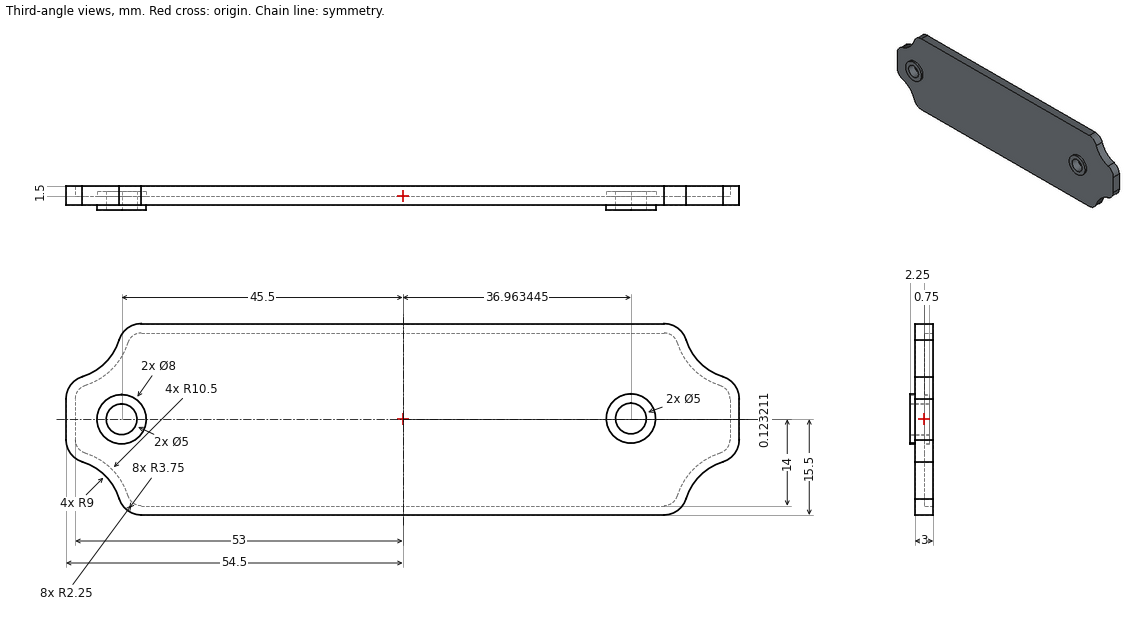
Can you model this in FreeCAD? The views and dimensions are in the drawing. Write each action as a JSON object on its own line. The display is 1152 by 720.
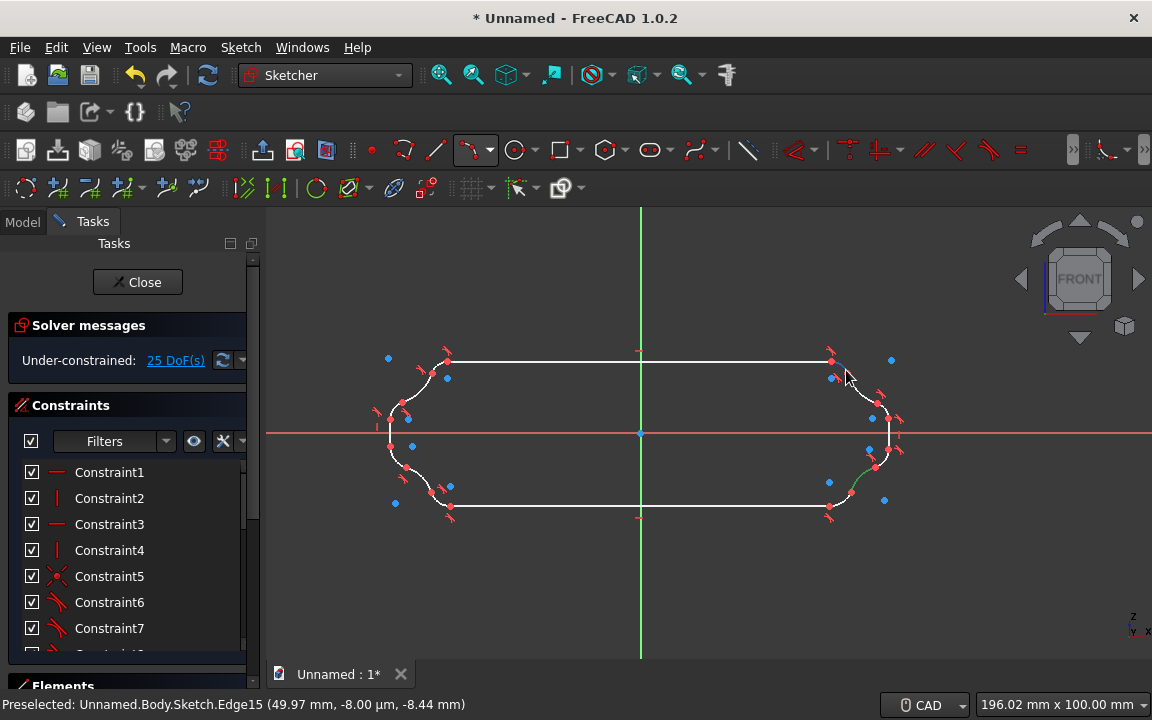
{"action": "scroll", "coordinate": [838, 505], "scroll_direction": "up", "scroll_amount": 3}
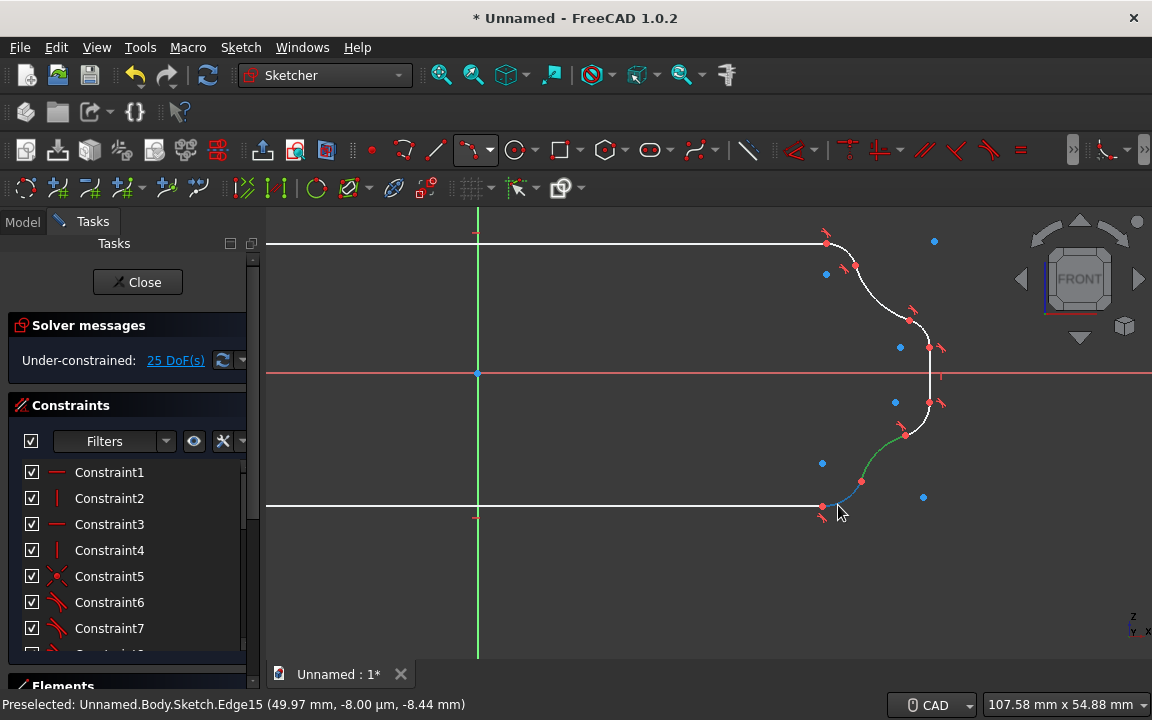
{"action": "left_click", "coordinate": [837, 504]}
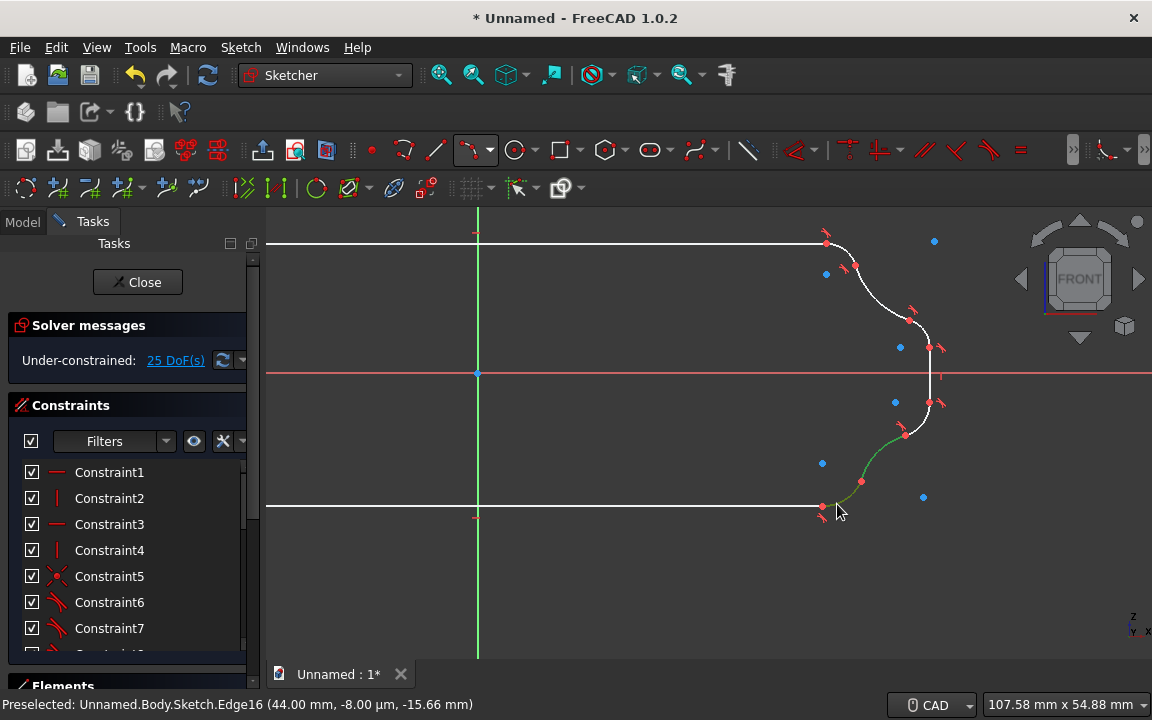
{"action": "left_click", "coordinate": [990, 150]}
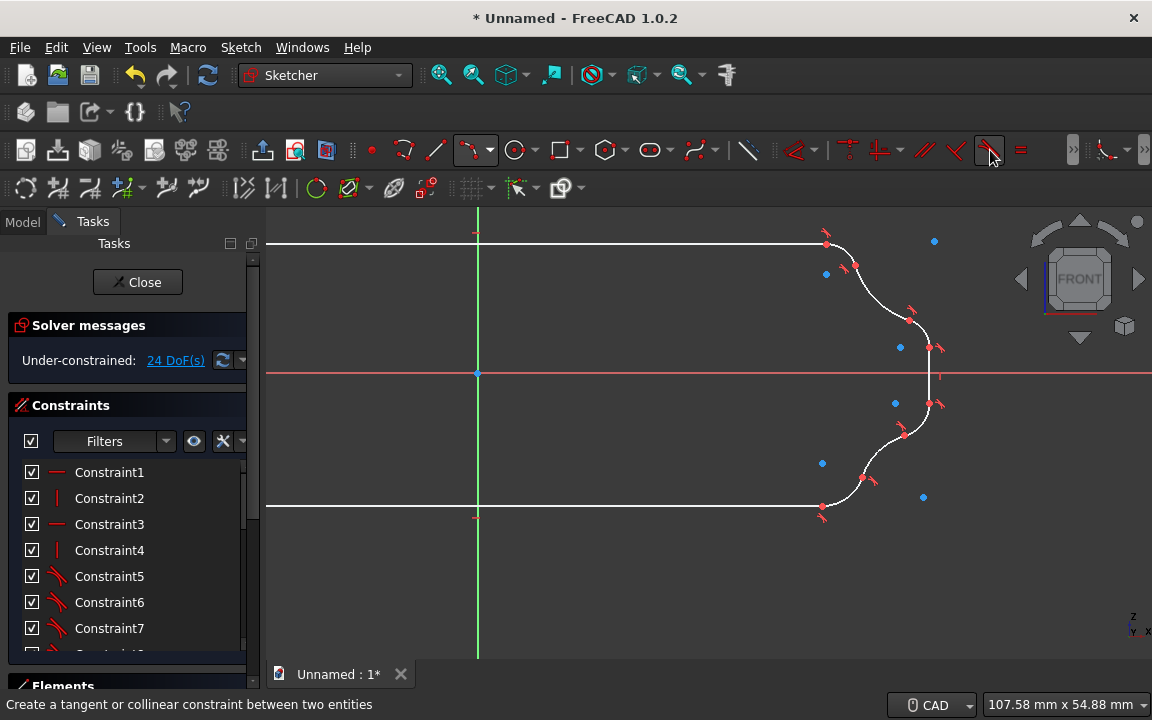
{"action": "scroll", "coordinate": [838, 506], "scroll_direction": "down", "scroll_amount": 3}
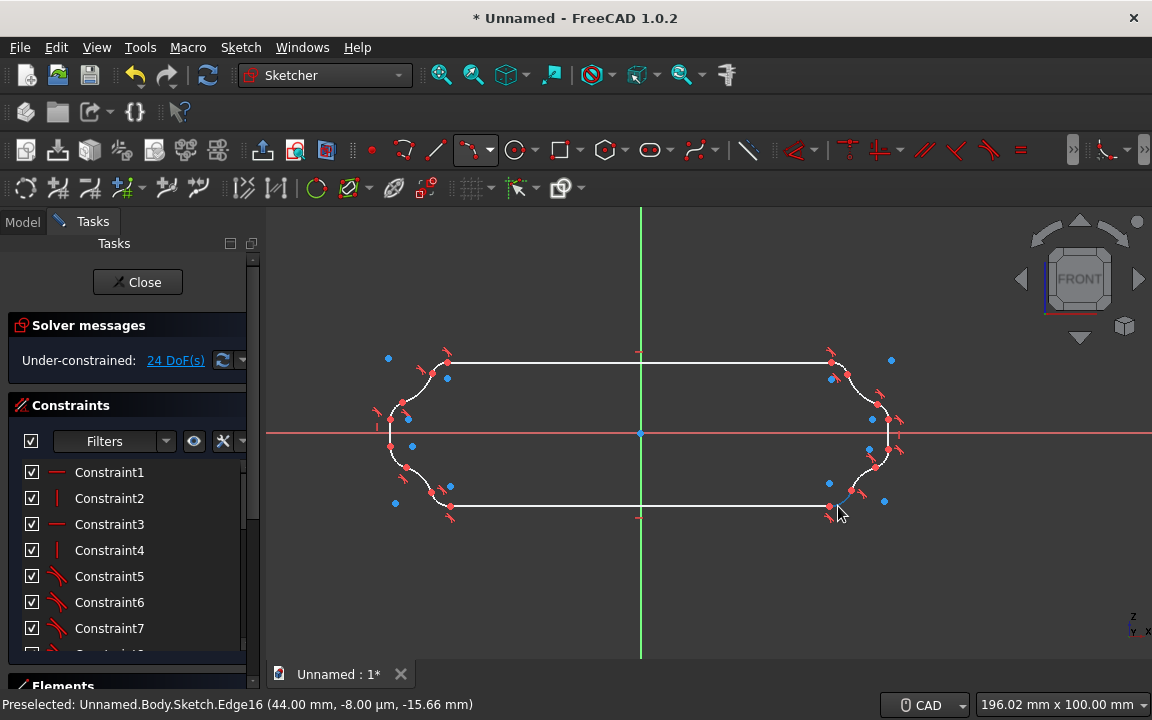
{"action": "scroll", "coordinate": [435, 499], "scroll_direction": "up", "scroll_amount": 4}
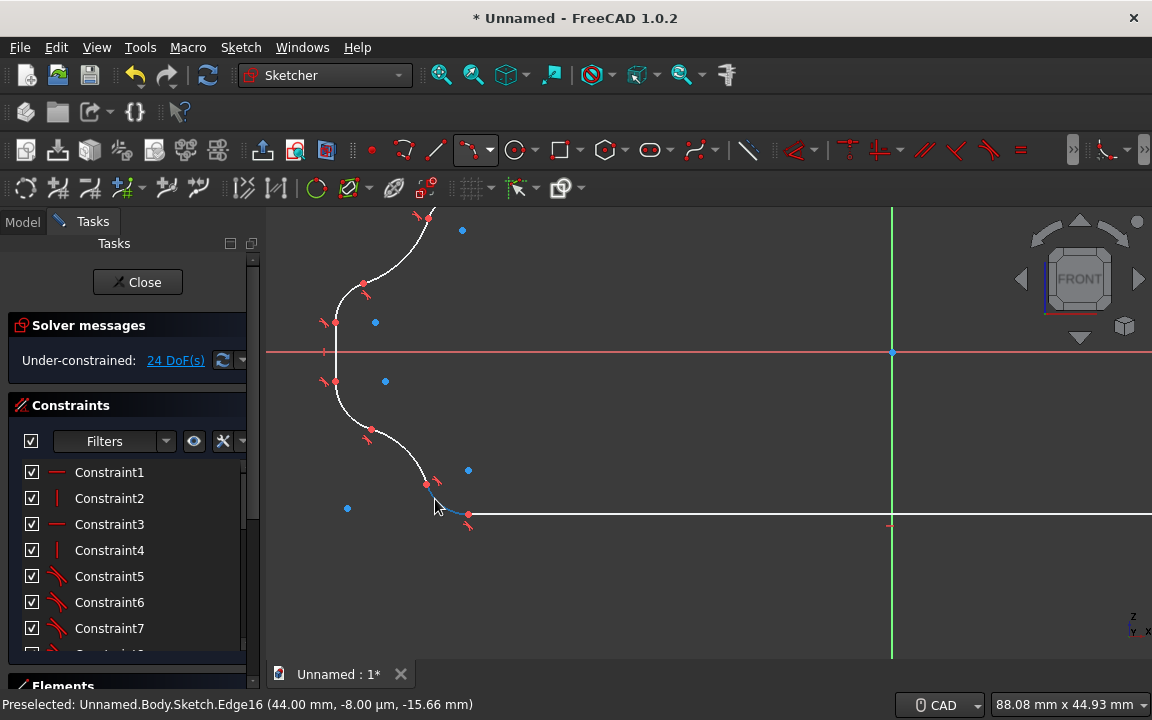
{"action": "left_click", "coordinate": [435, 498]}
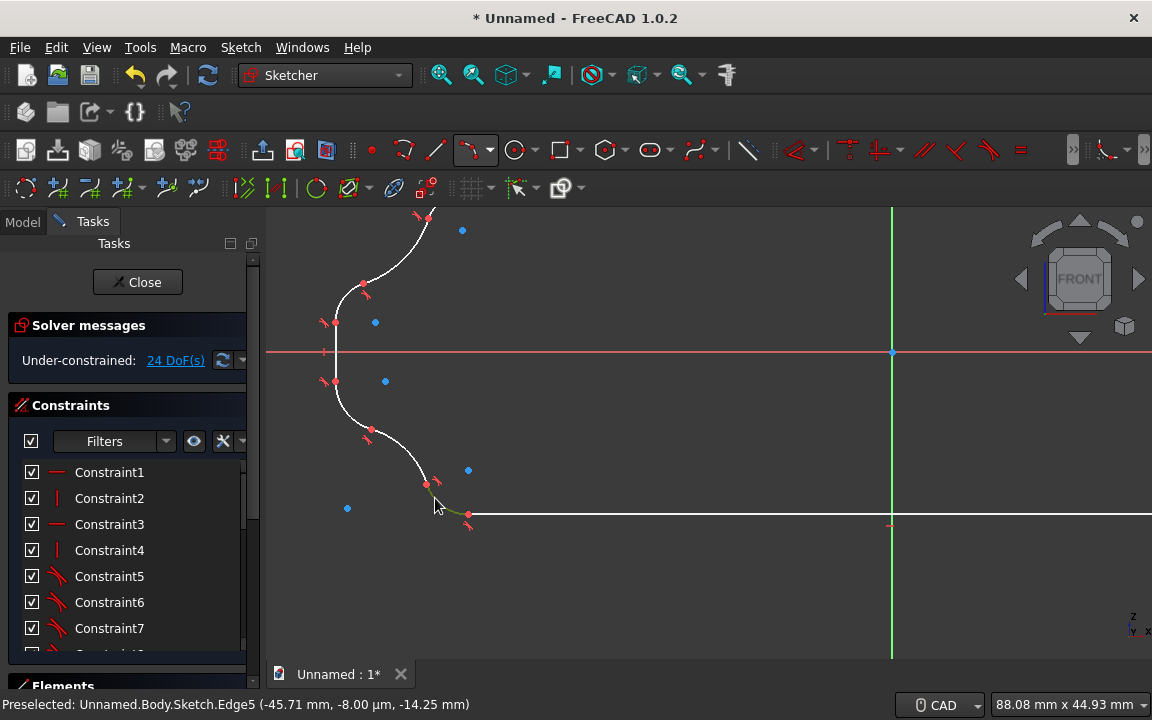
{"action": "left_click", "coordinate": [339, 400]}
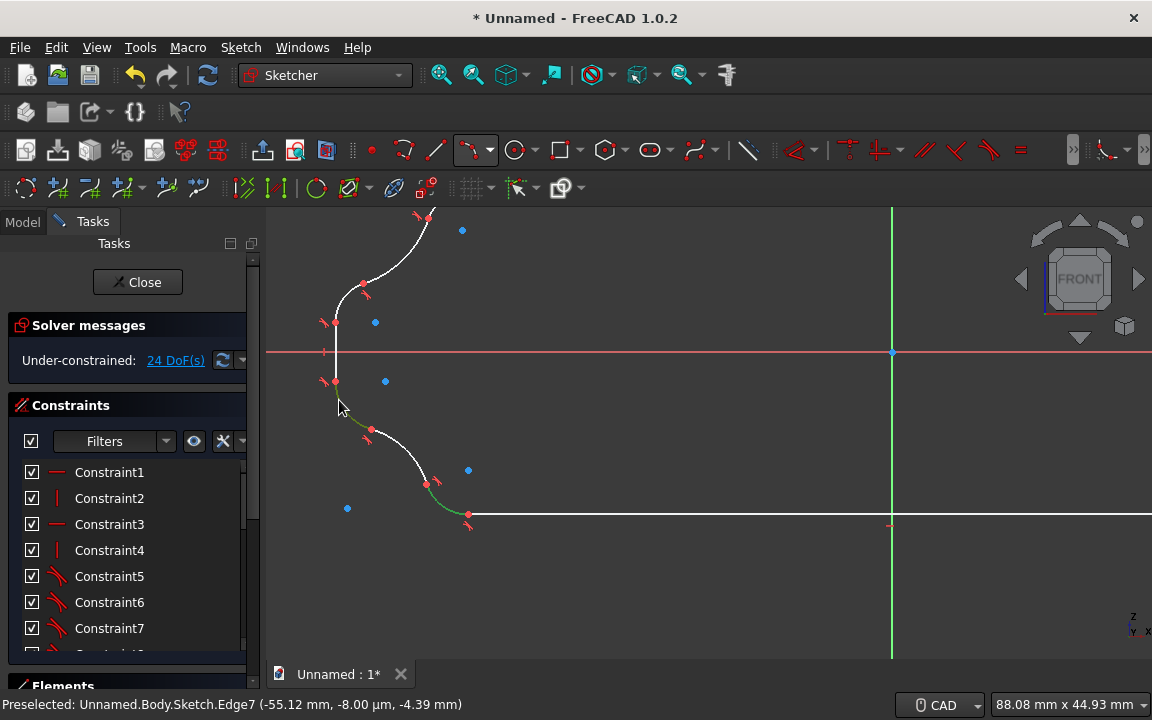
{"action": "left_click", "coordinate": [350, 291]}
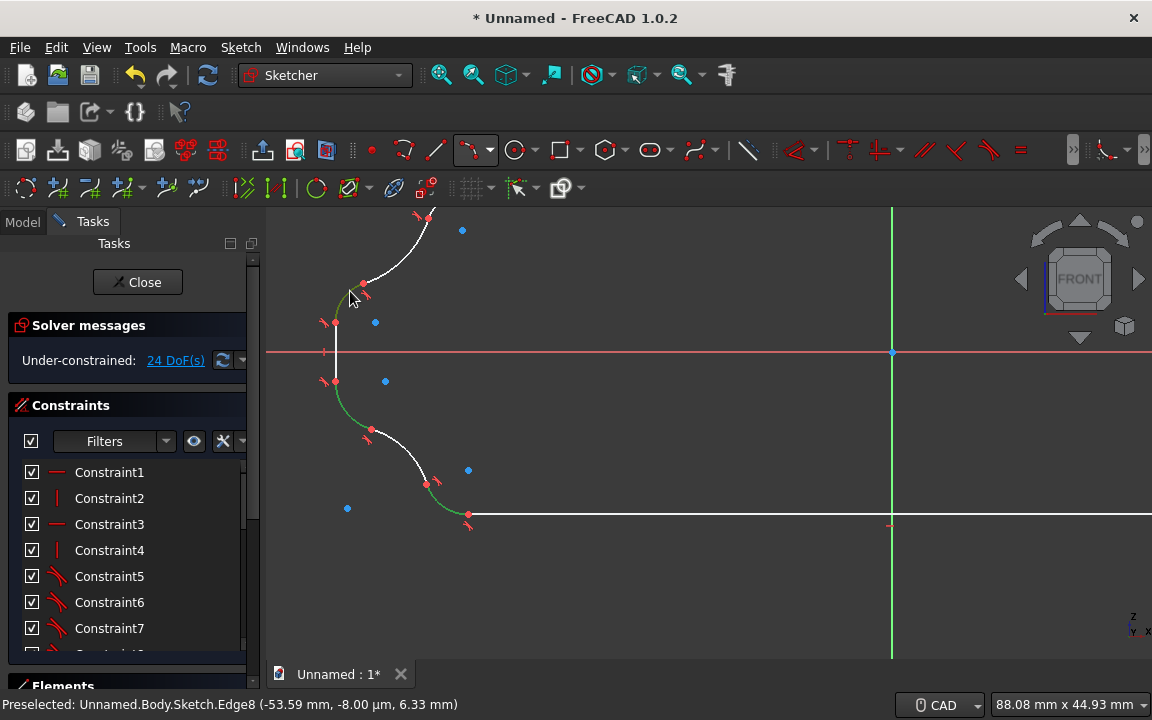
{"action": "scroll", "coordinate": [435, 499], "scroll_direction": "down", "scroll_amount": 4}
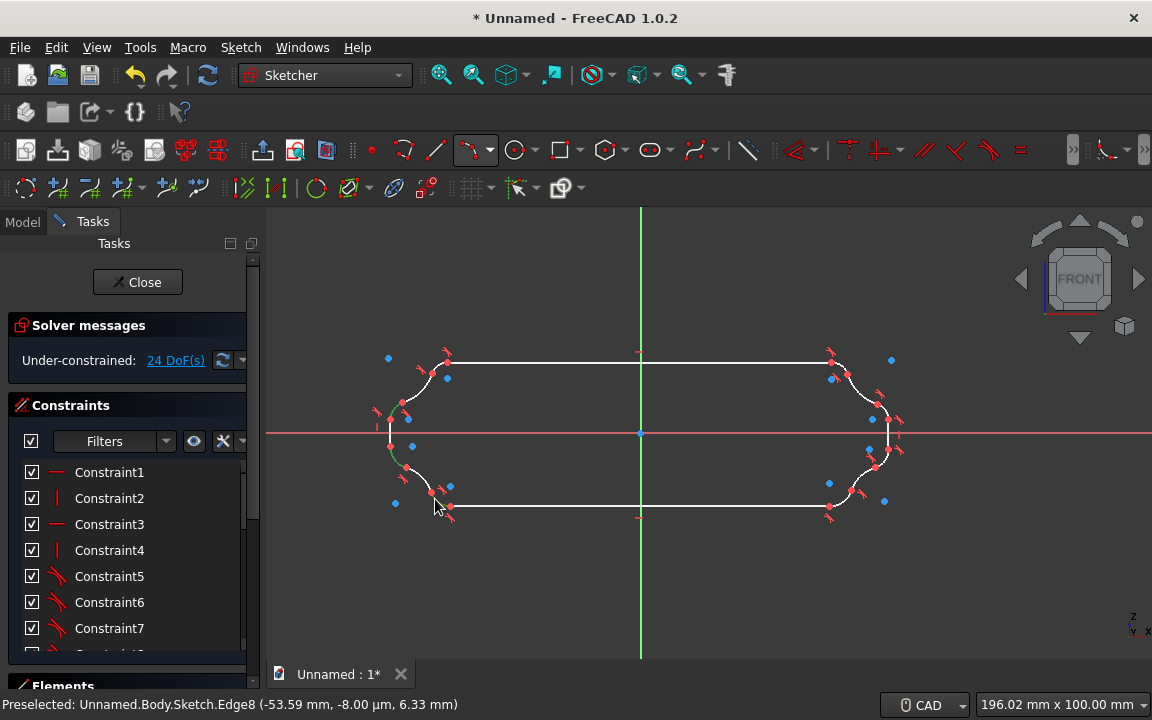
{"action": "scroll", "coordinate": [442, 364], "scroll_direction": "up", "scroll_amount": 5}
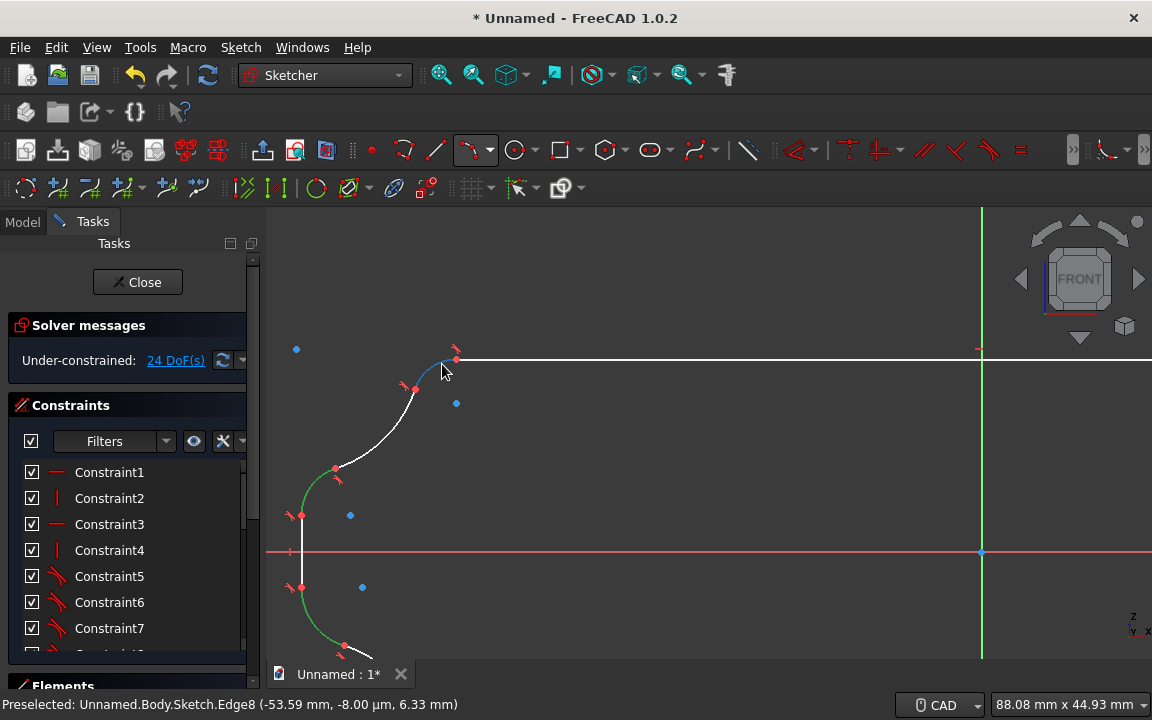
{"action": "left_click", "coordinate": [440, 363]}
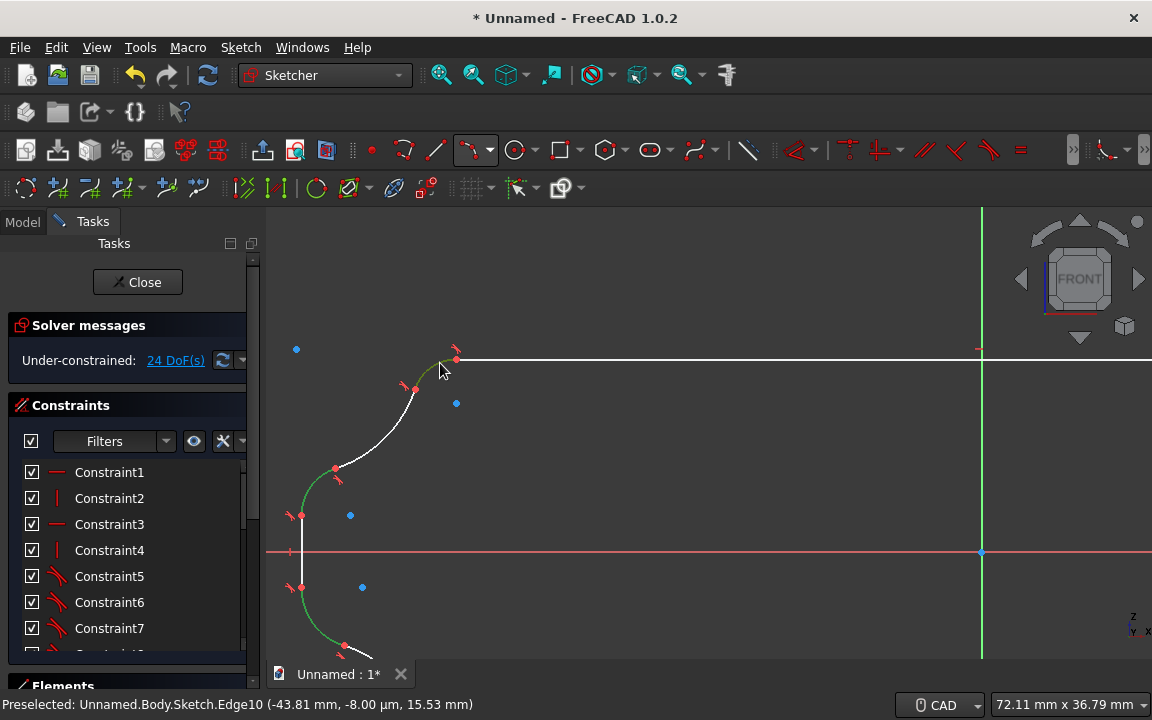
{"action": "scroll", "coordinate": [442, 364], "scroll_direction": "down", "scroll_amount": 5}